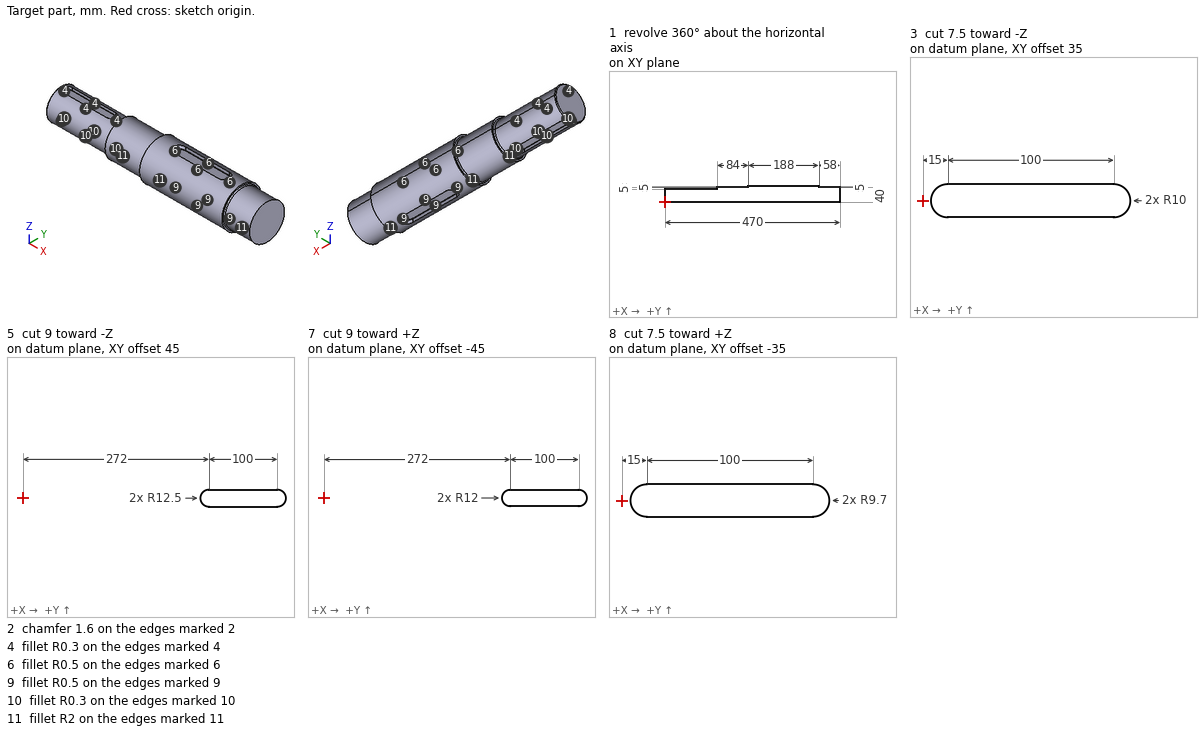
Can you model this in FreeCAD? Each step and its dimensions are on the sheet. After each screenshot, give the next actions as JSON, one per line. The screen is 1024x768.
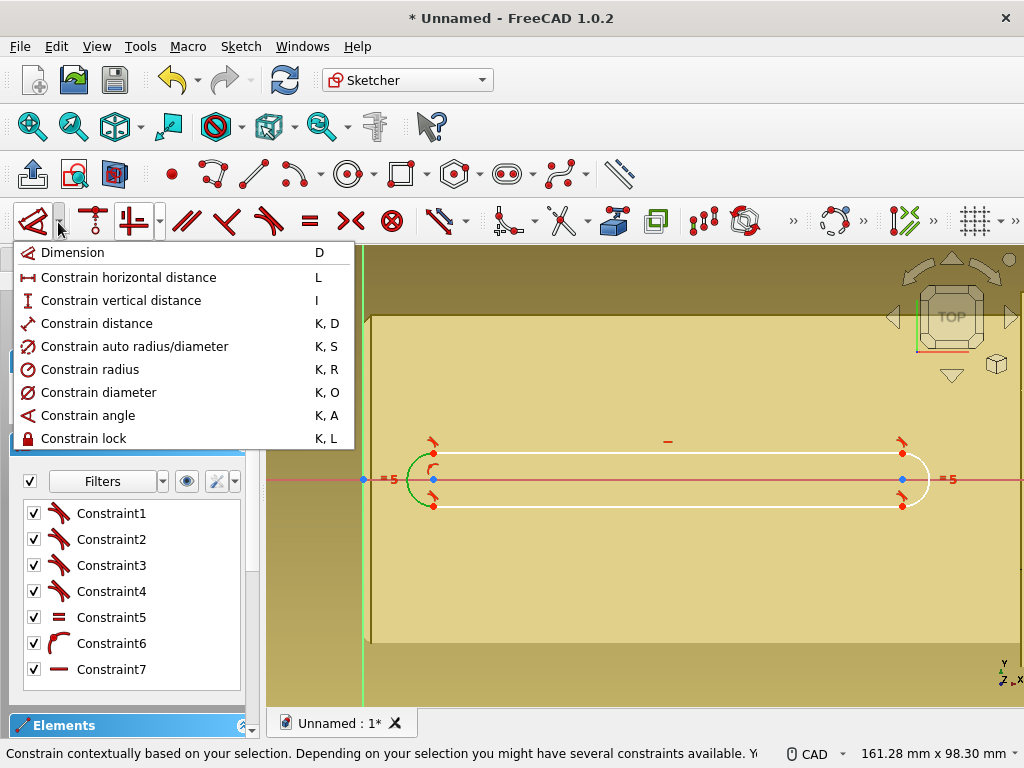
{"action": "left_click", "coordinate": [184, 370]}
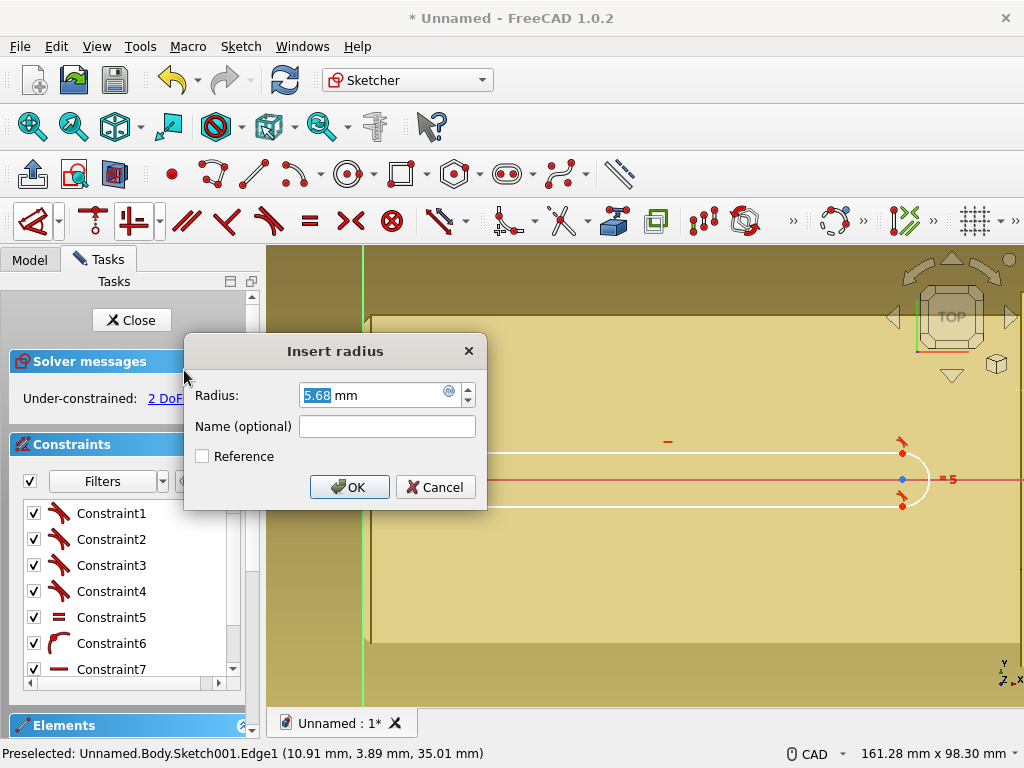
{"action": "type", "text": "10"}
{"action": "key", "text": "Return"}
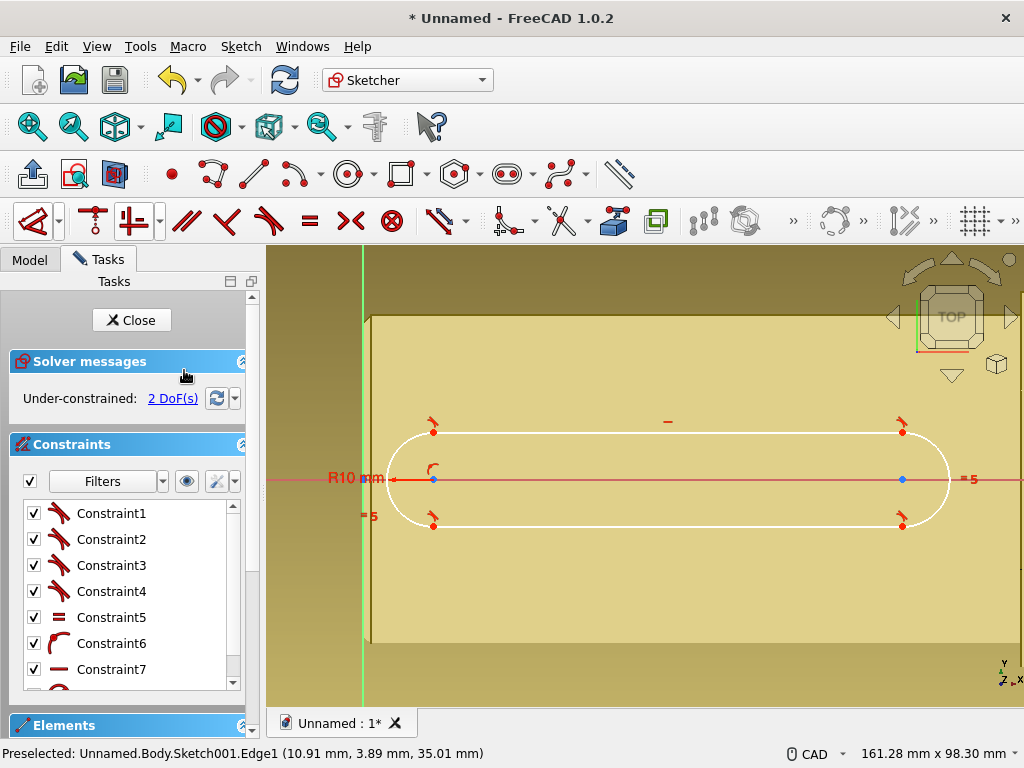
{"action": "left_click", "coordinate": [575, 433]}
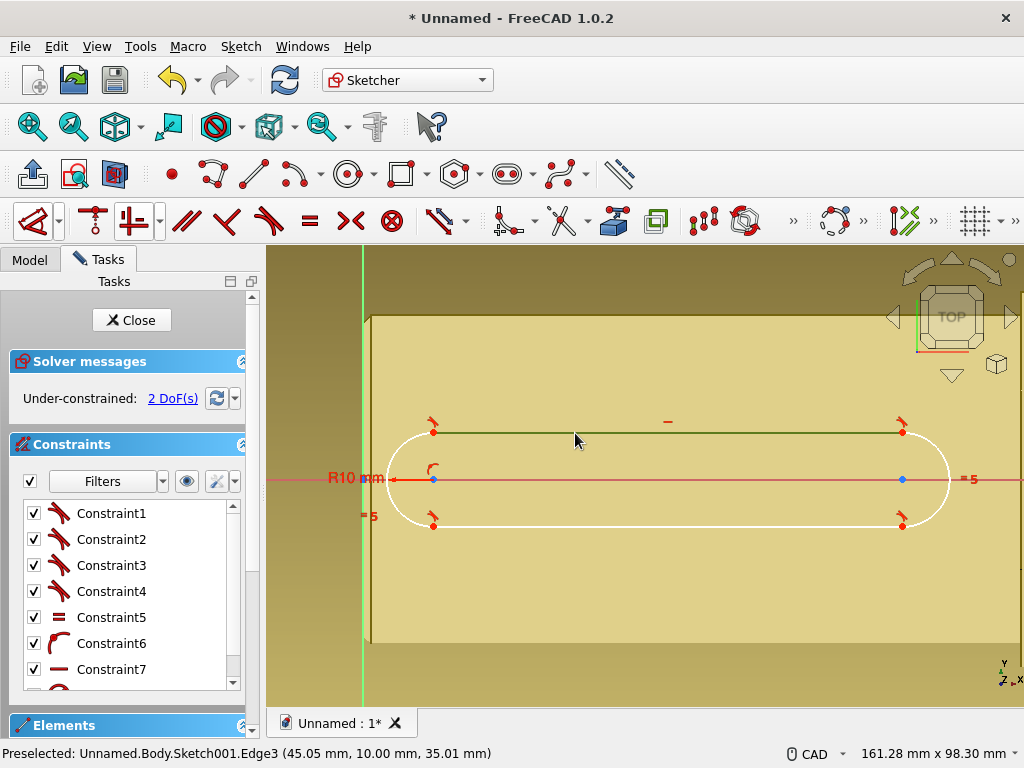
{"action": "left_click", "coordinate": [58, 222]}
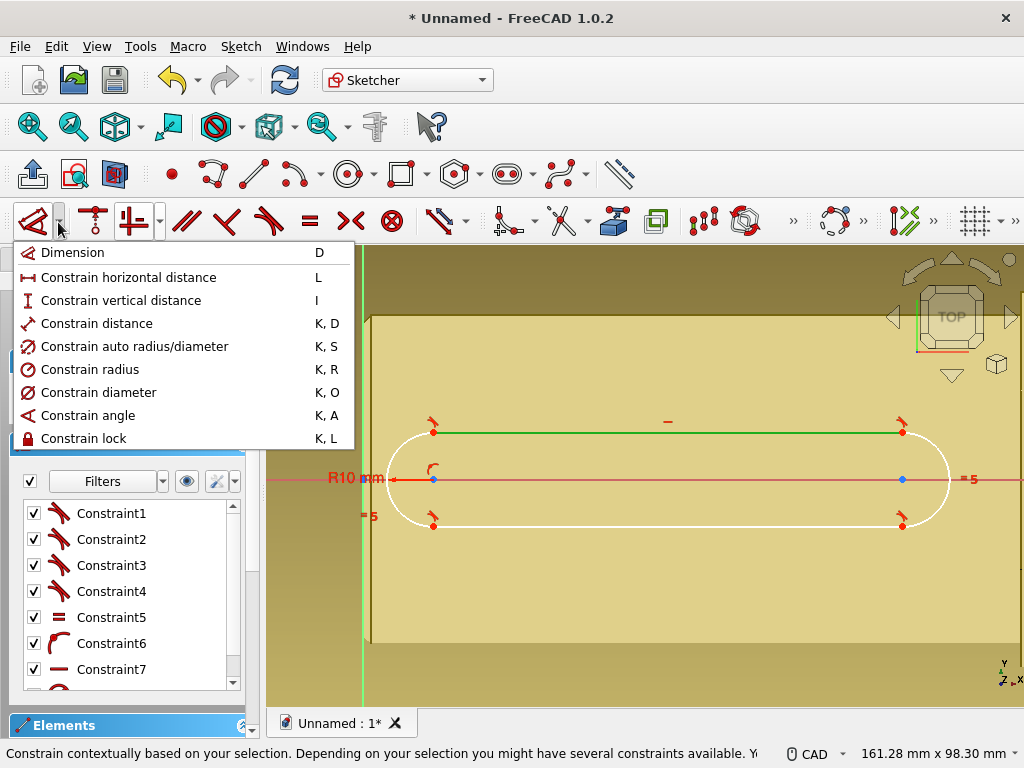
{"action": "left_click", "coordinate": [184, 278]}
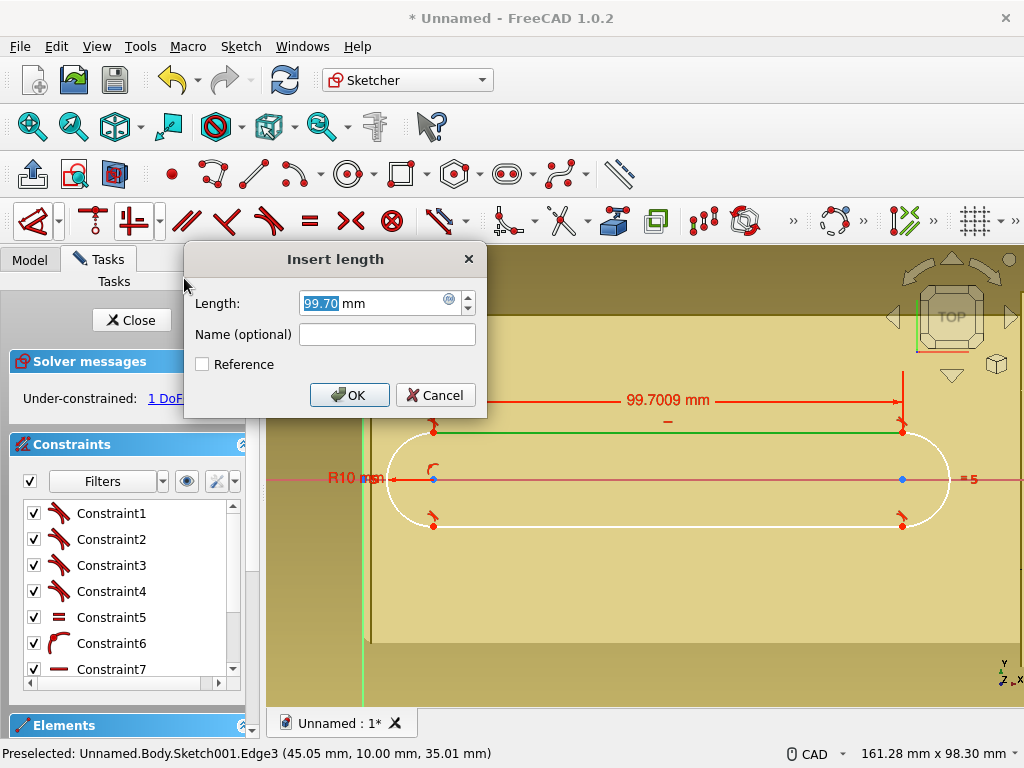
{"action": "type", "text": "100"}
{"action": "key", "text": "Return"}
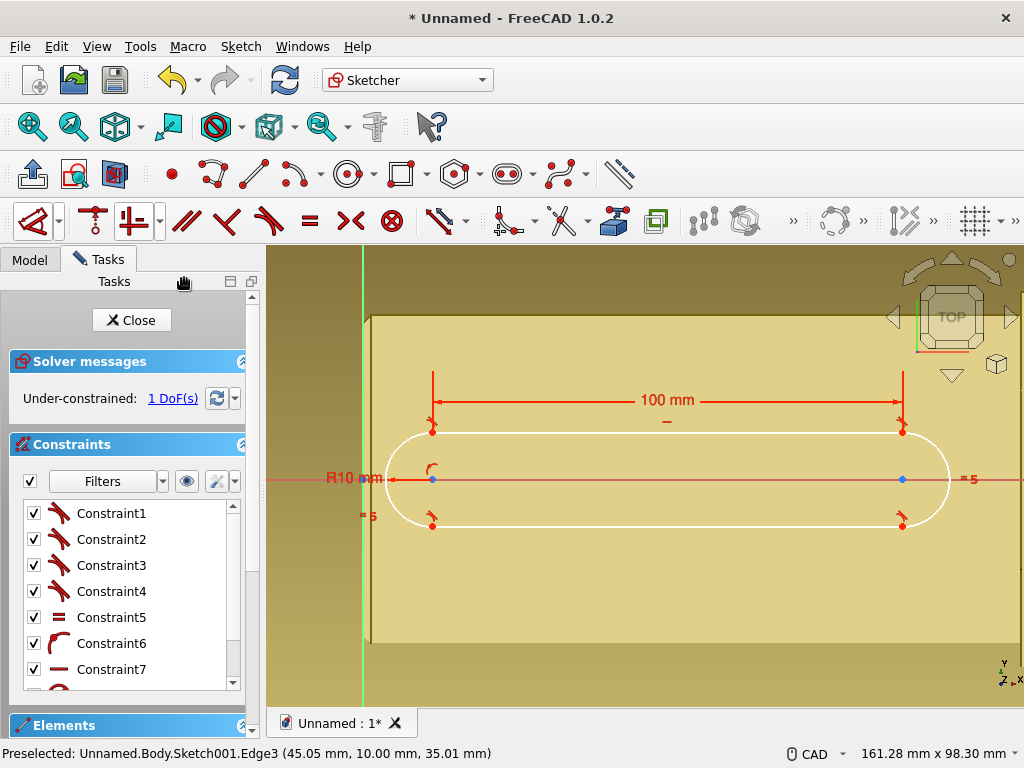
{"action": "left_click", "coordinate": [433, 433]}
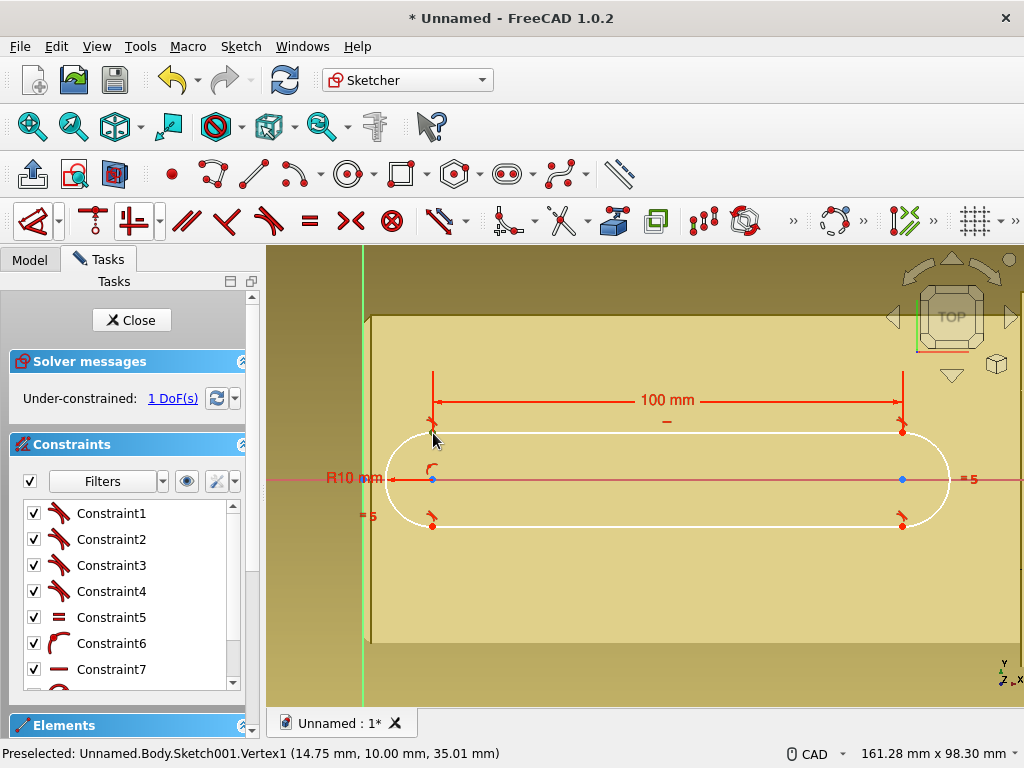
{"action": "left_click", "coordinate": [58, 222]}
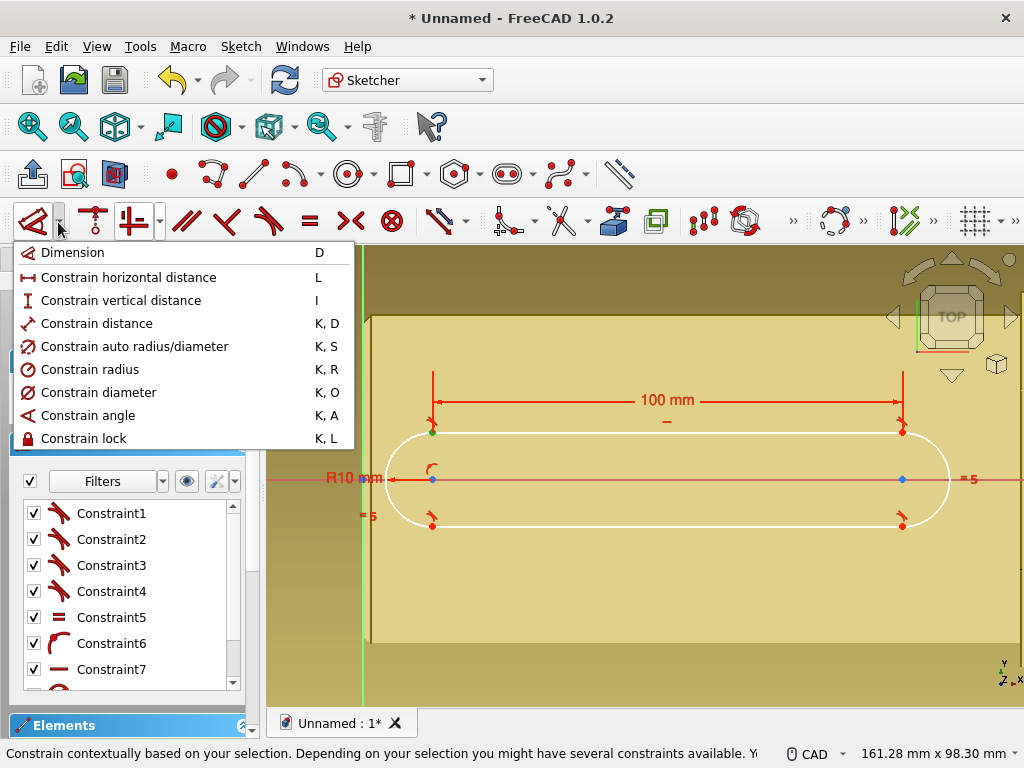
{"action": "left_click", "coordinate": [184, 278]}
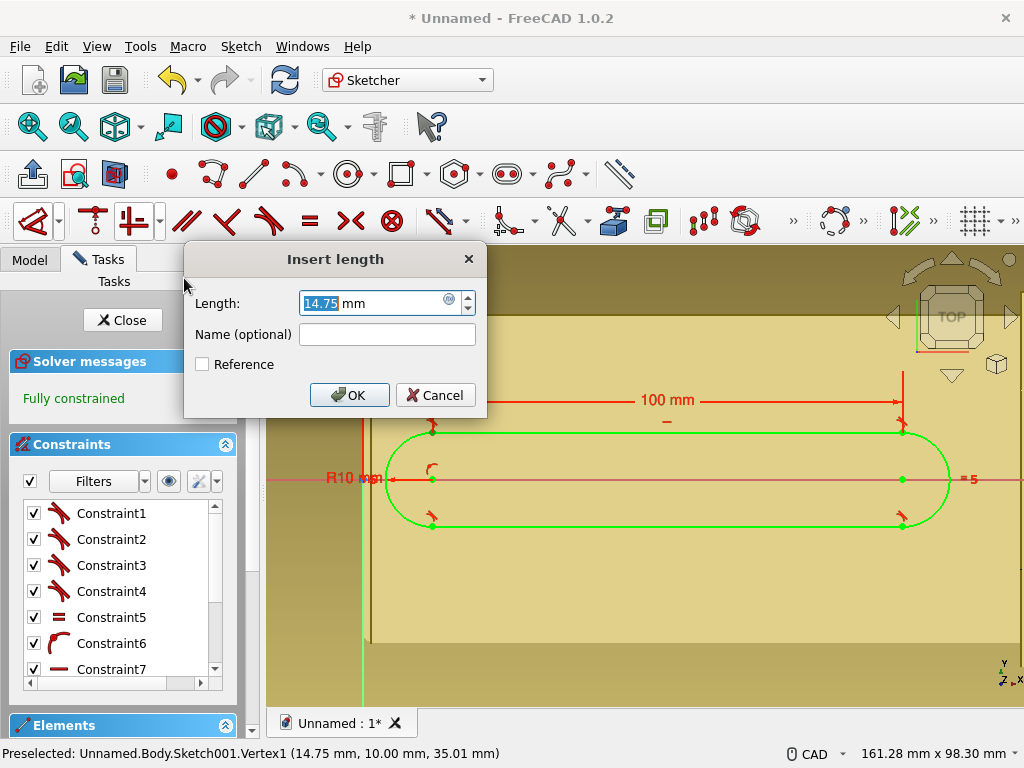
{"action": "type", "text": "15"}
{"action": "key", "text": "Return"}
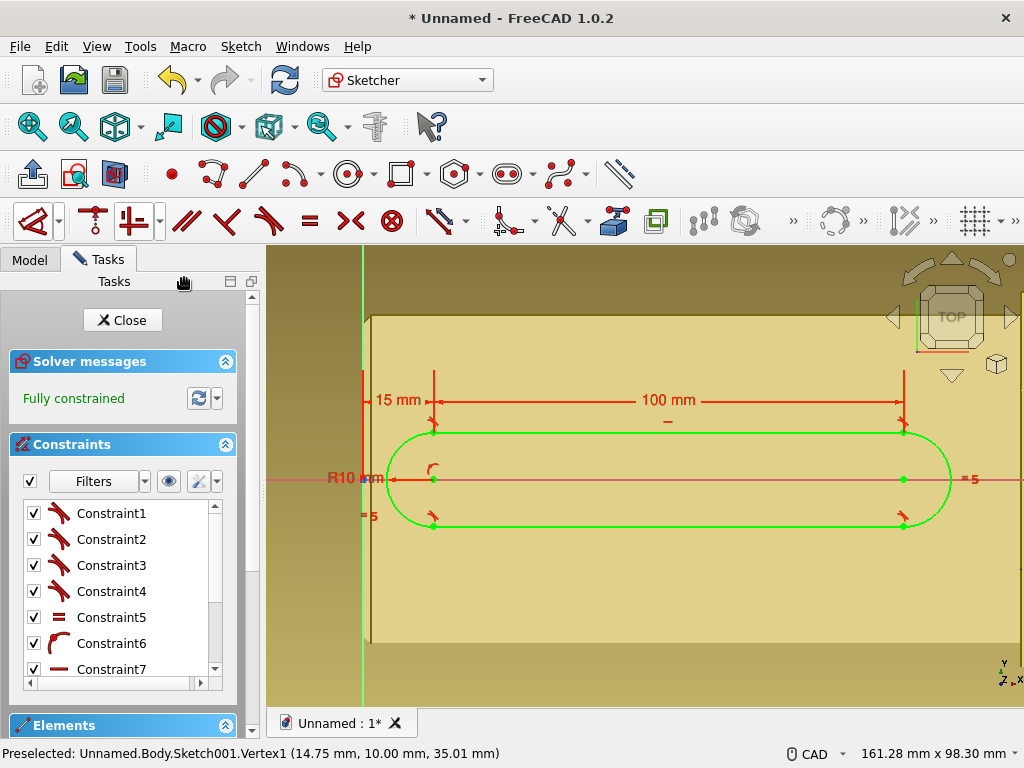
{"action": "left_click", "coordinate": [123, 320]}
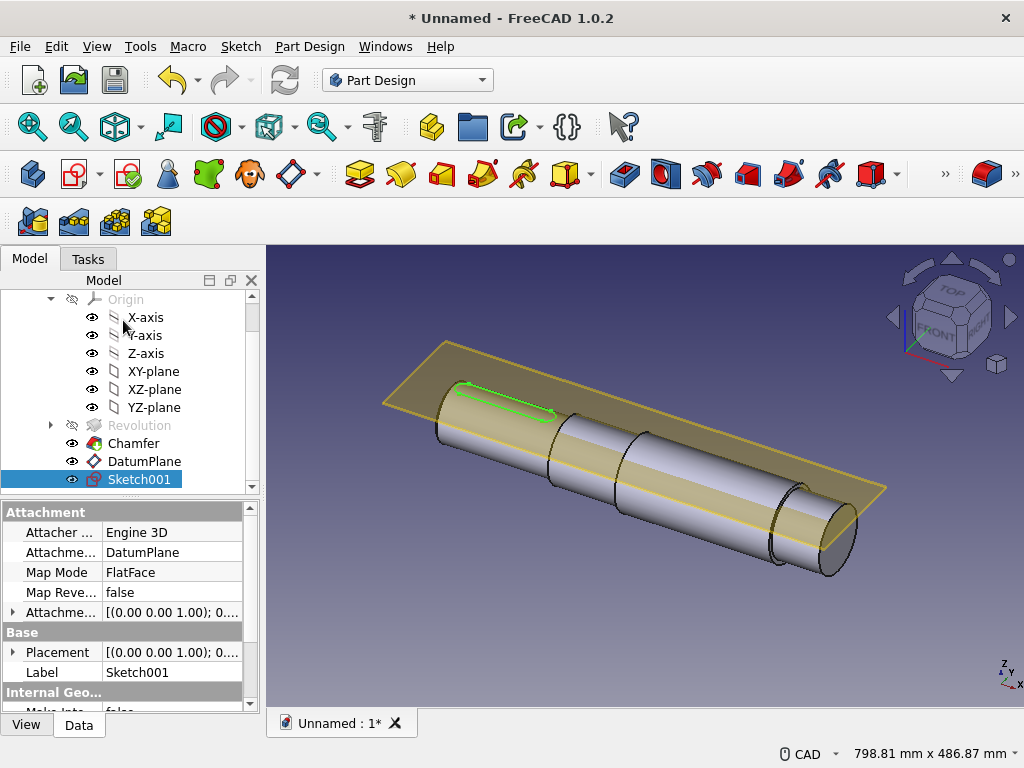
{"action": "left_click", "coordinate": [625, 174]}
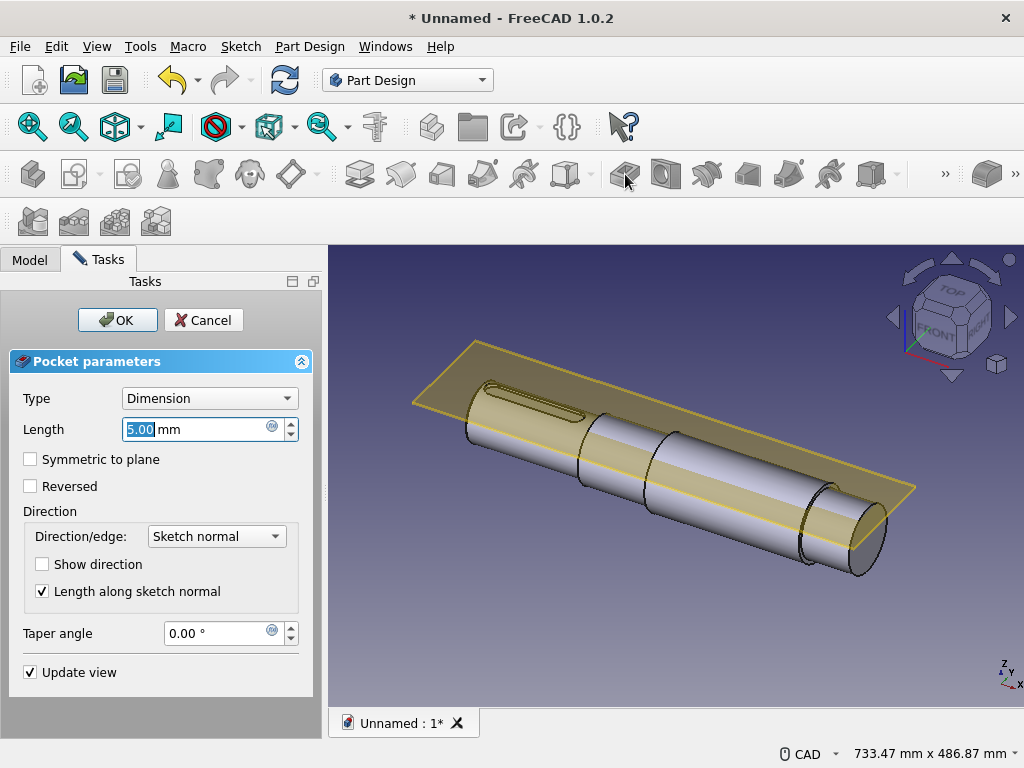
{"action": "type", "text": "7.5"}
{"action": "key", "text": "Tab"}